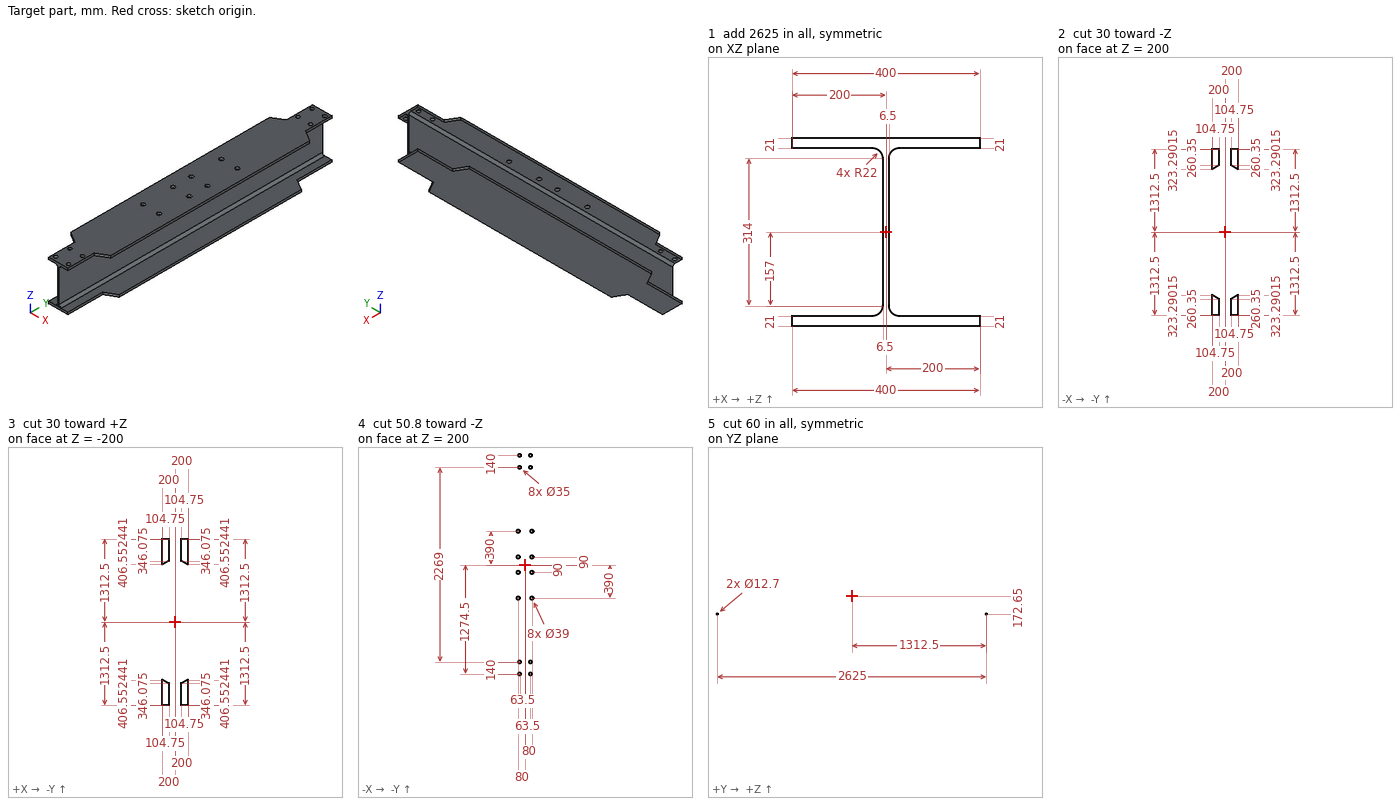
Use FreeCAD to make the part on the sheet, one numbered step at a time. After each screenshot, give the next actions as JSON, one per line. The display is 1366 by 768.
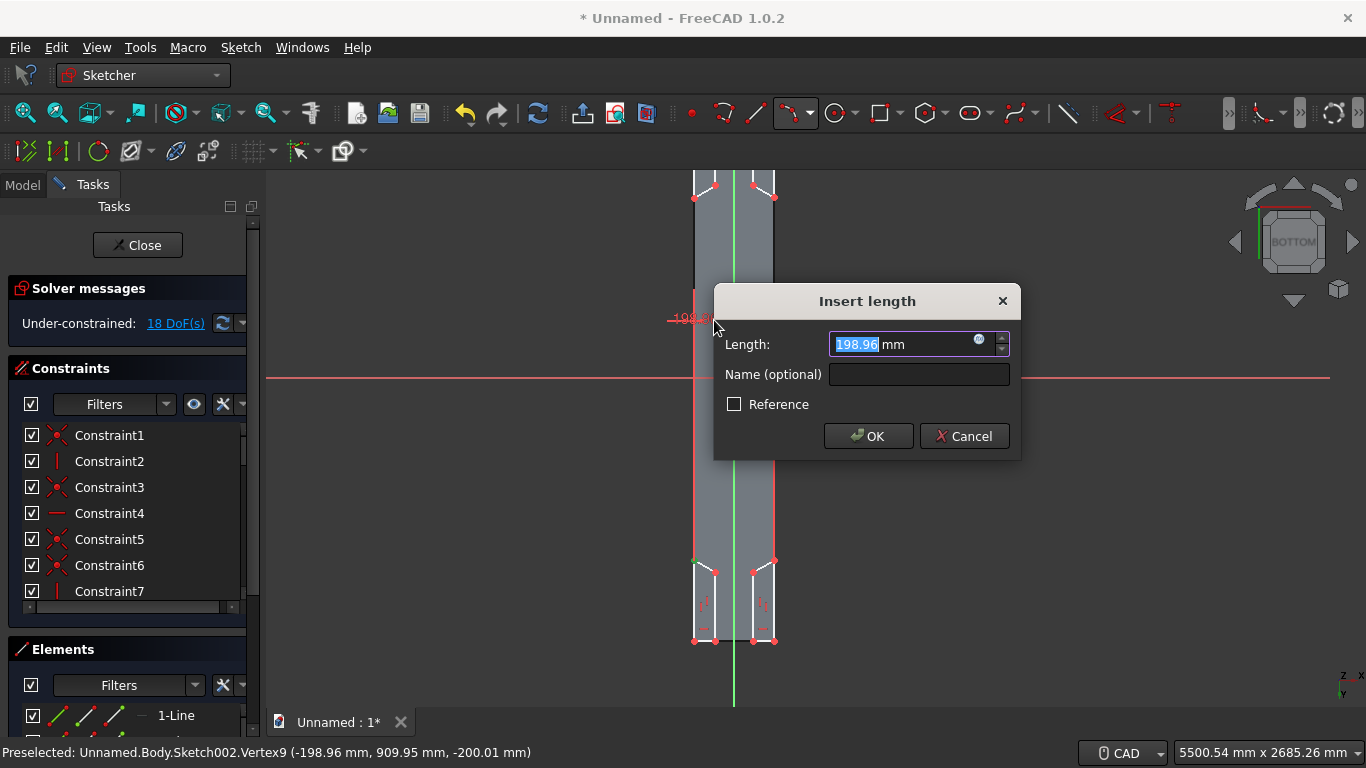
{"action": "type", "text": "200"}
{"action": "key", "text": "Return"}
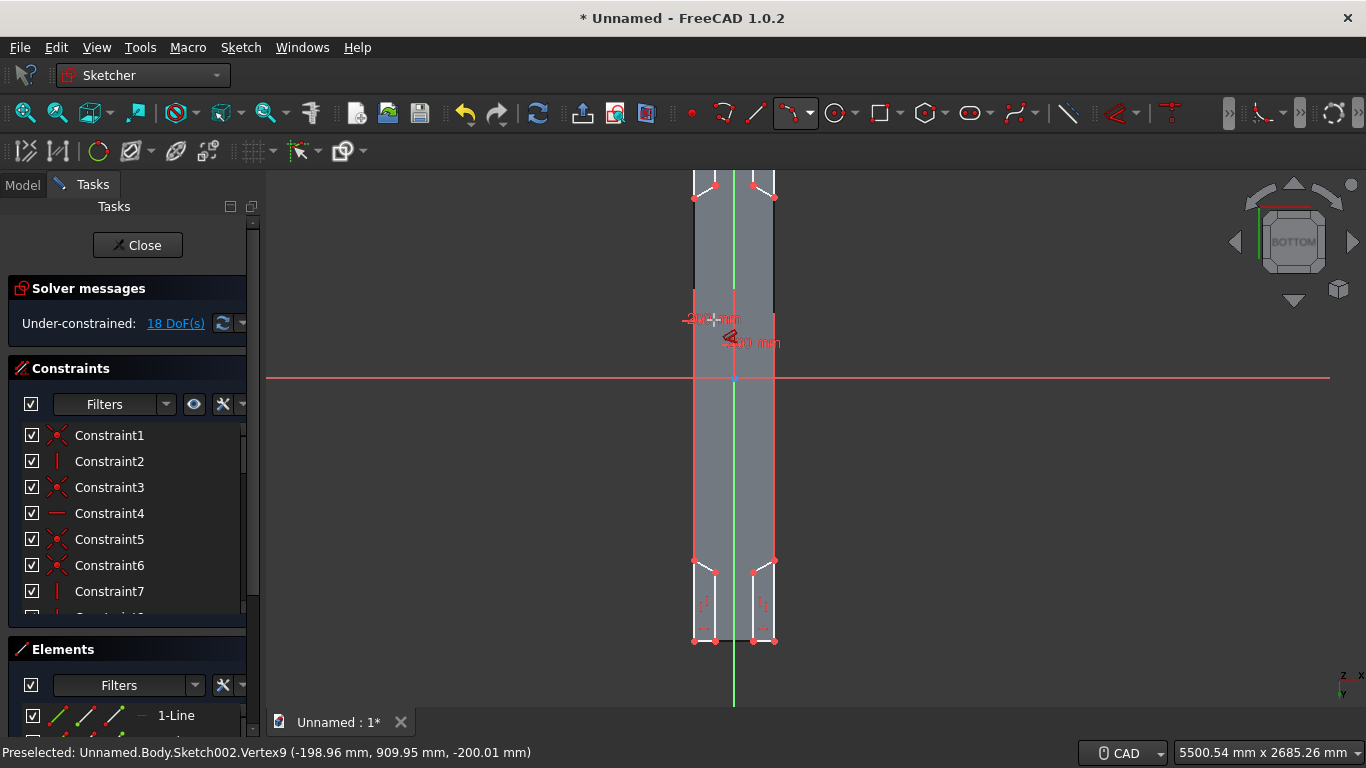
{"action": "left_click", "coordinate": [694, 198]}
{"action": "left_click", "coordinate": [714, 412]}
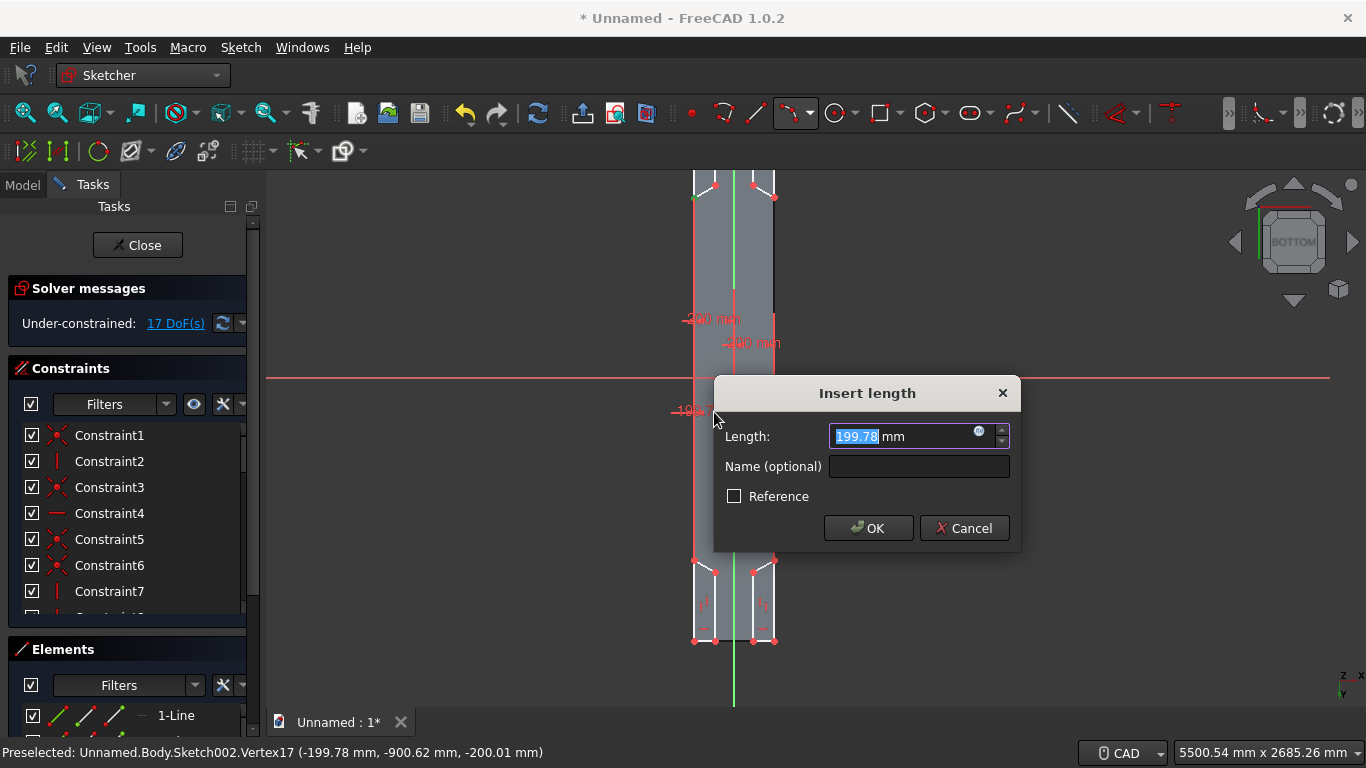
{"action": "type", "text": "200"}
{"action": "key", "text": "Return"}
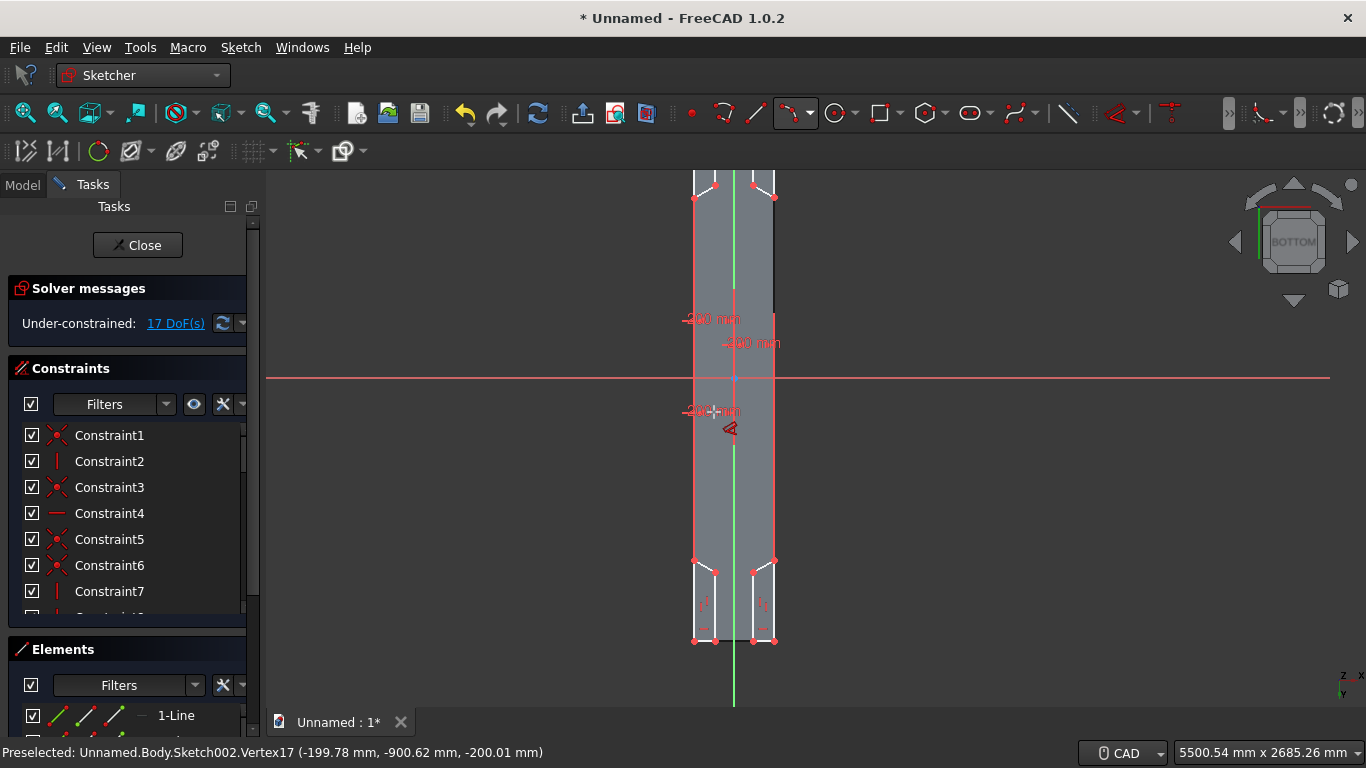
{"action": "scroll", "coordinate": [774, 561], "scroll_direction": "down", "scroll_amount": 2}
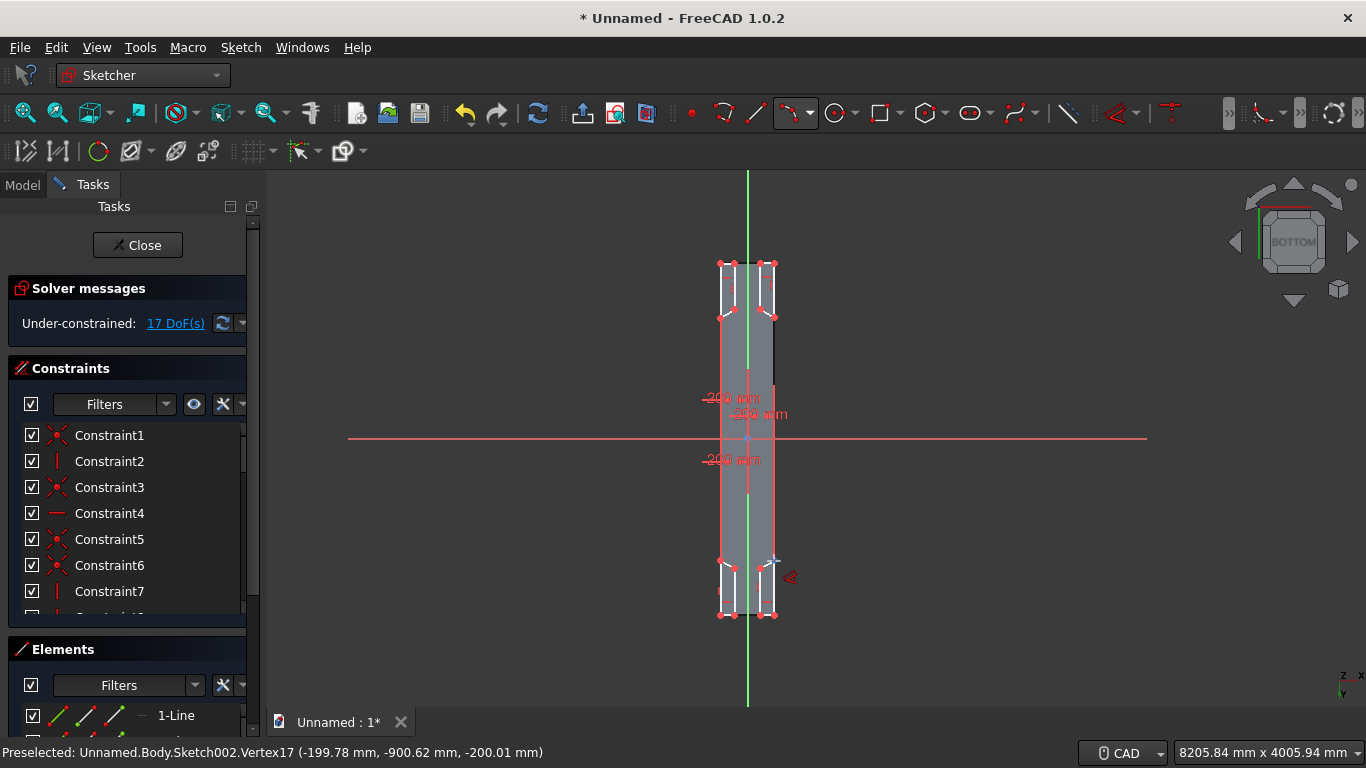
{"action": "scroll", "coordinate": [774, 318], "scroll_direction": "up", "scroll_amount": 2}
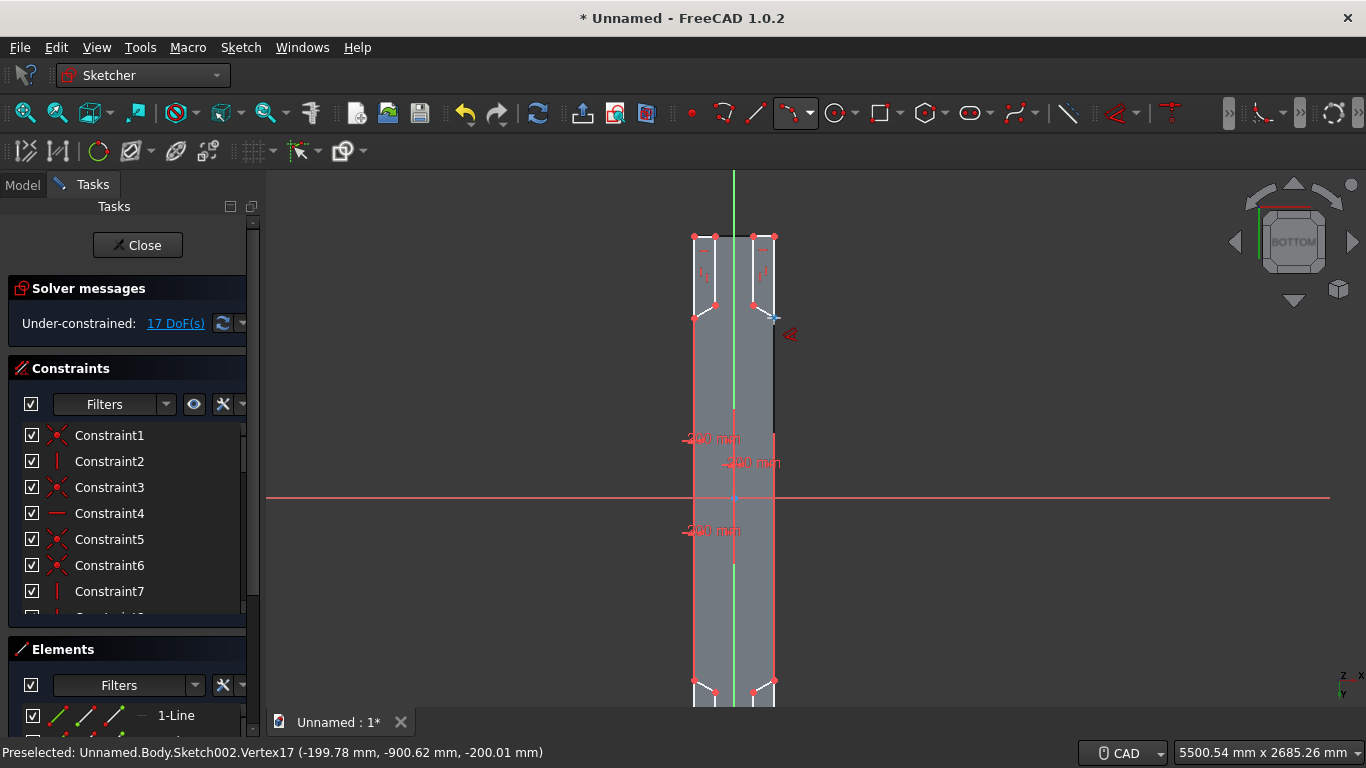
{"action": "left_click", "coordinate": [774, 317]}
{"action": "left_click", "coordinate": [754, 556]}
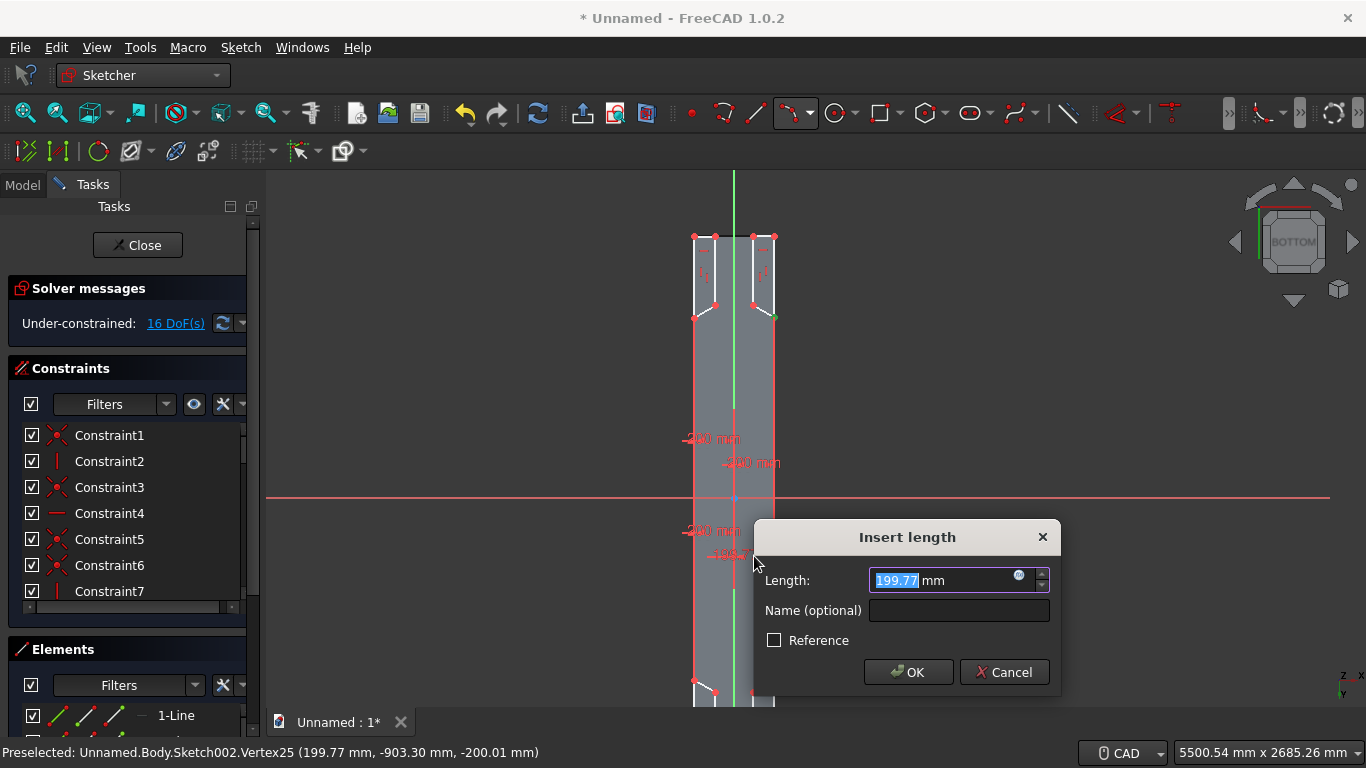
{"action": "type", "text": "200"}
{"action": "key", "text": "Return"}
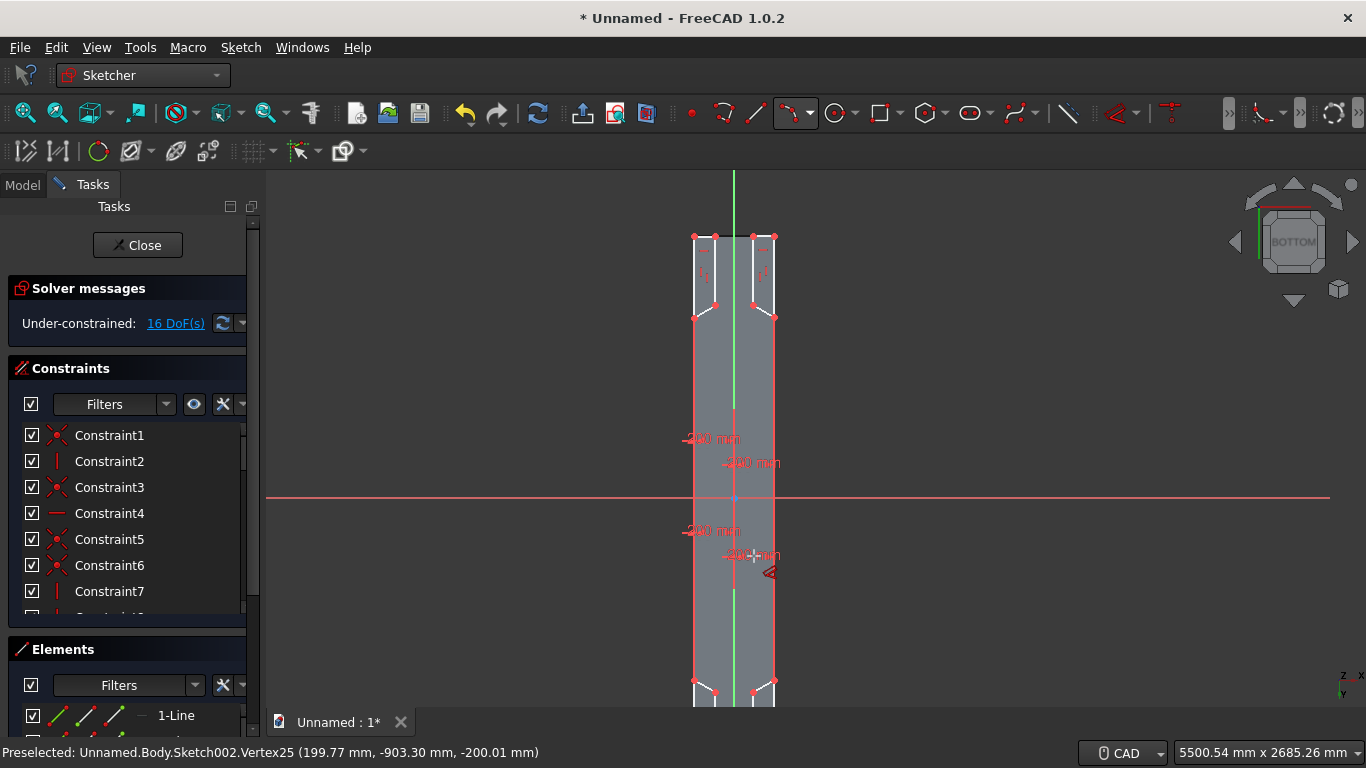
{"action": "scroll", "coordinate": [774, 317], "scroll_direction": "down", "scroll_amount": 2}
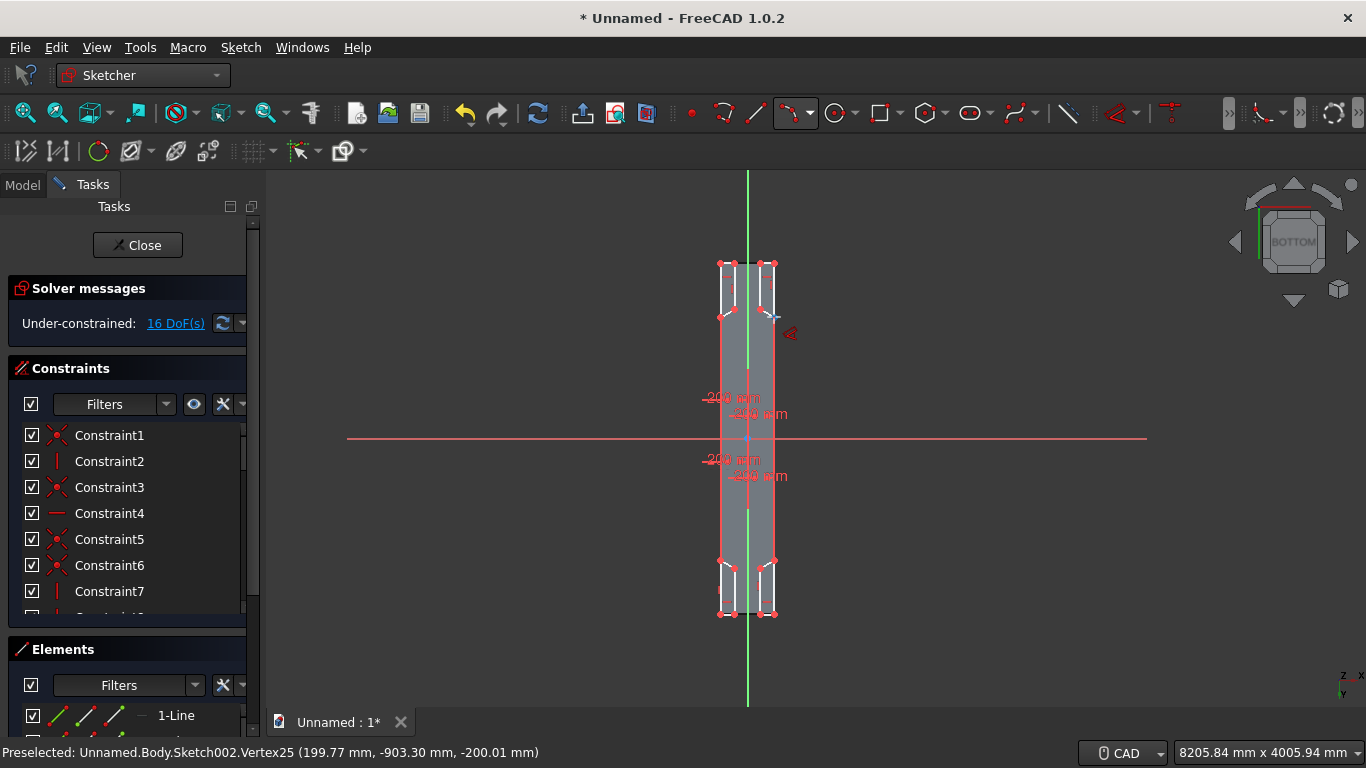
{"action": "scroll", "coordinate": [767, 615], "scroll_direction": "up", "scroll_amount": 6}